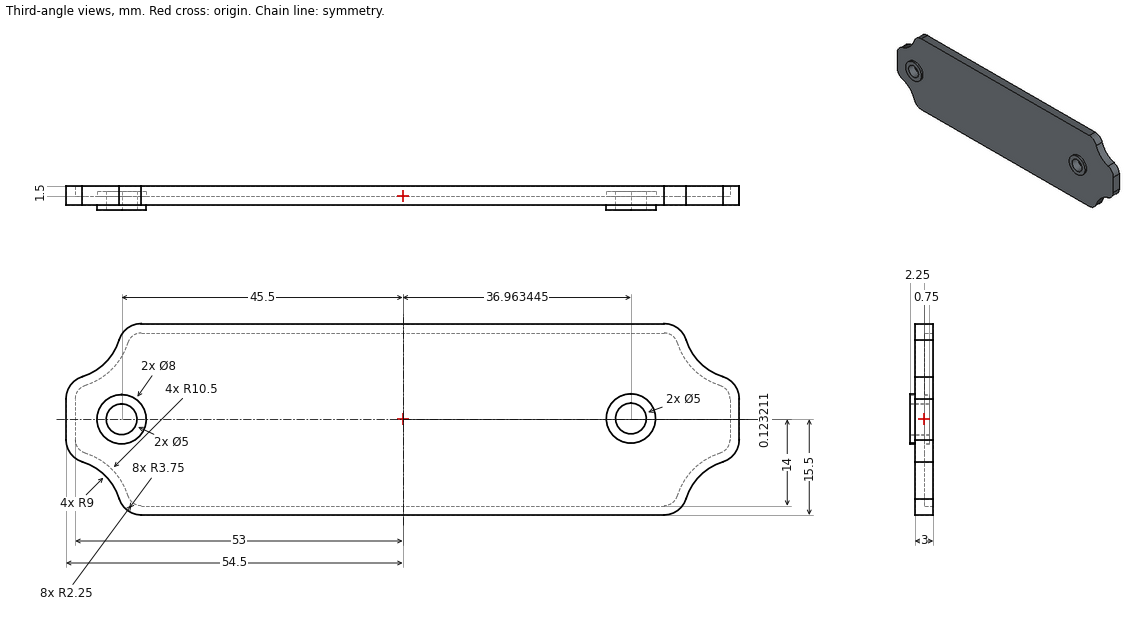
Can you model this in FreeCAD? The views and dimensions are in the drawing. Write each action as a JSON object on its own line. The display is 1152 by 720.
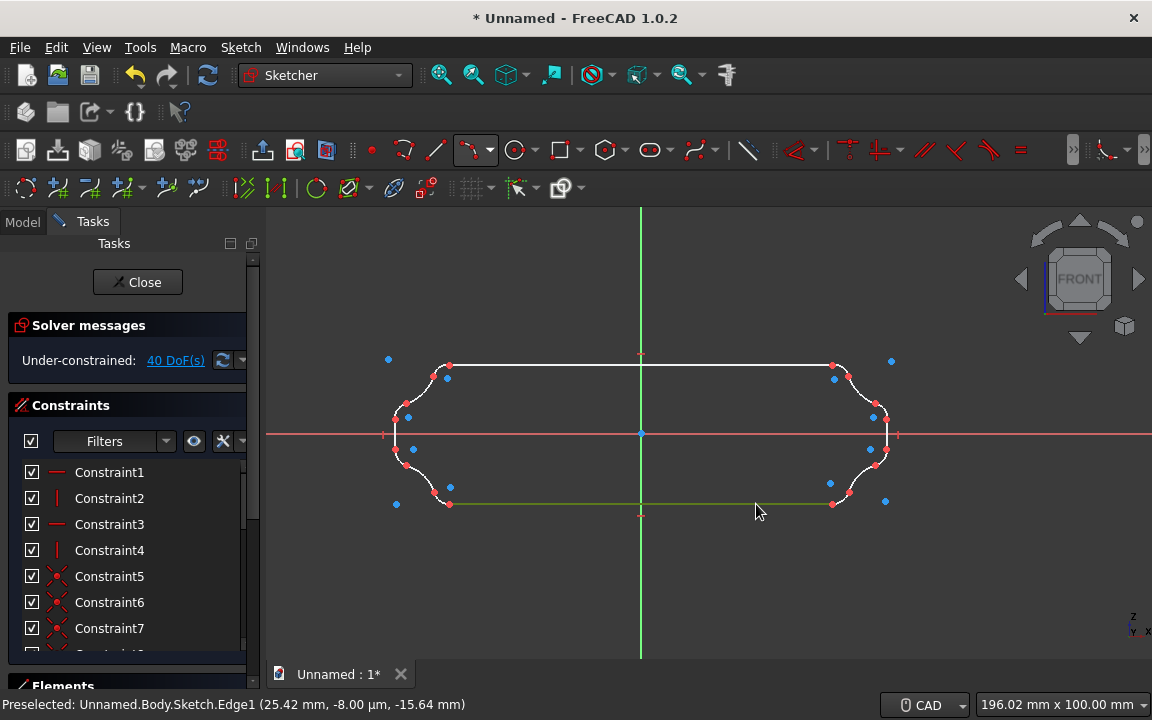
{"action": "scroll", "coordinate": [440, 501], "scroll_direction": "up", "scroll_amount": 2}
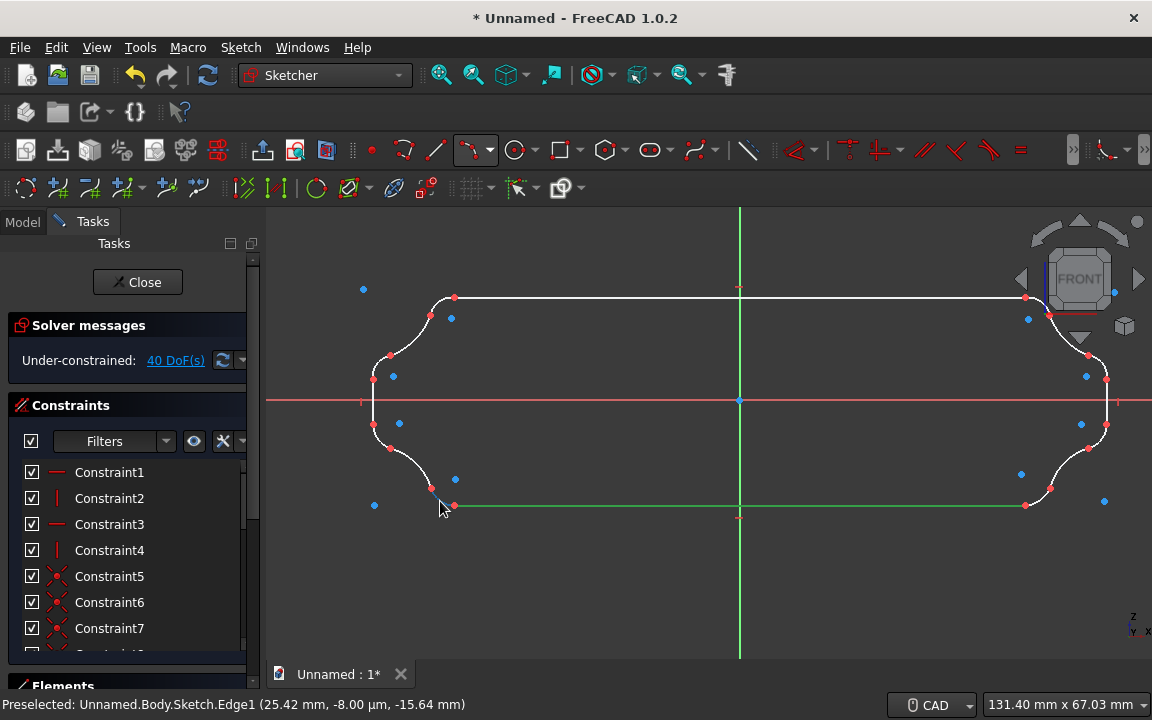
{"action": "left_click", "coordinate": [440, 501]}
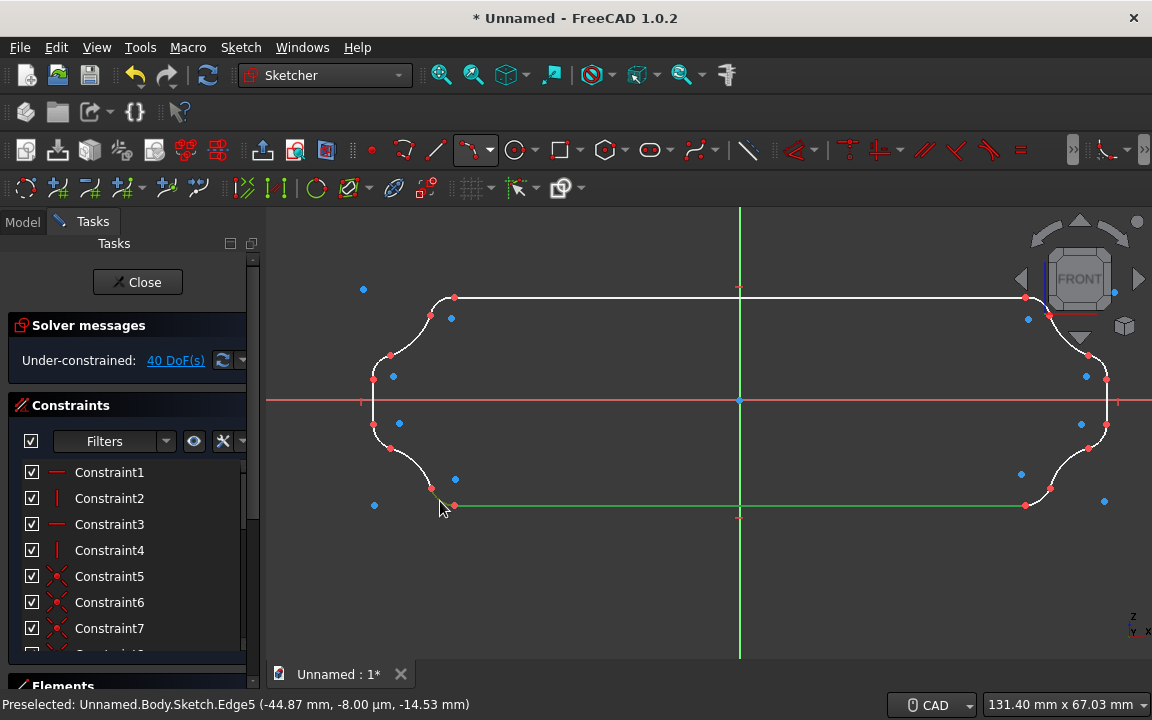
{"action": "left_click", "coordinate": [990, 150]}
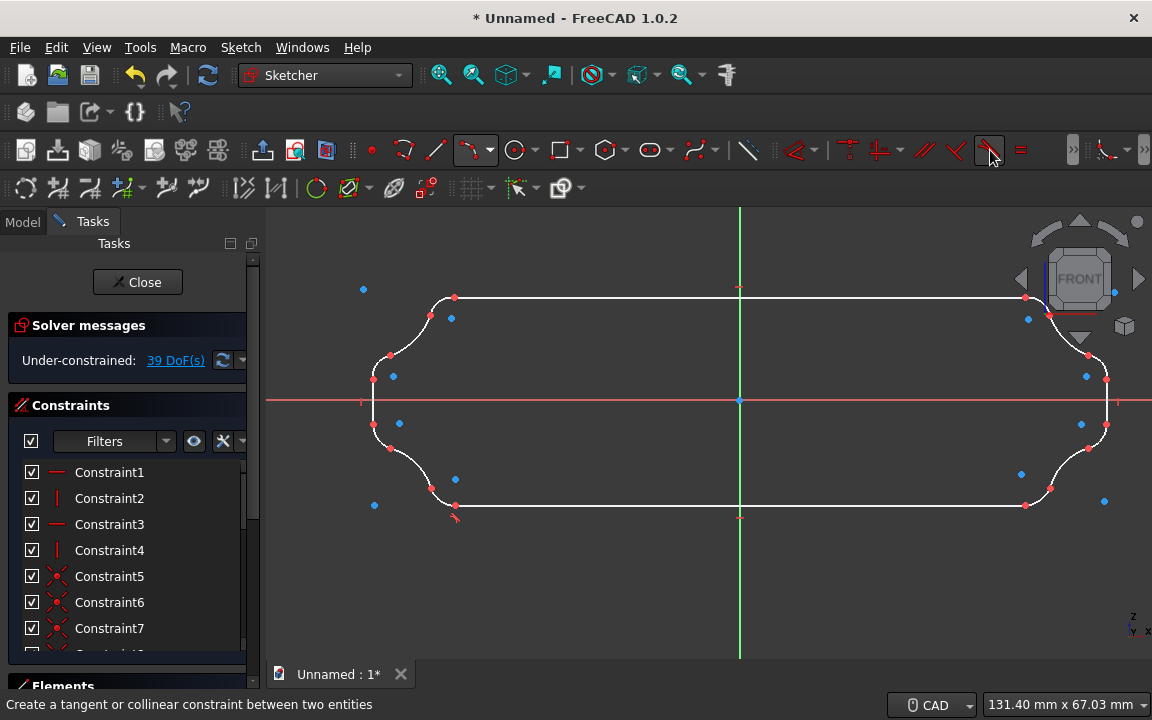
{"action": "left_click", "coordinate": [854, 506]}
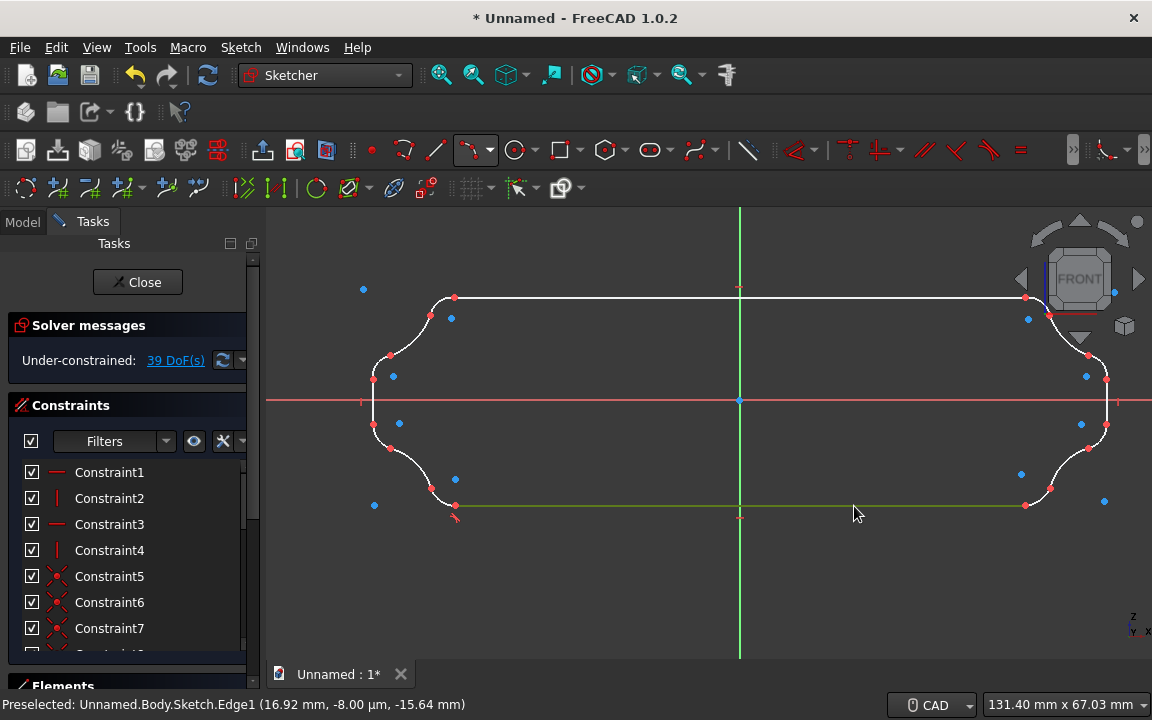
{"action": "scroll", "coordinate": [438, 499], "scroll_direction": "down", "scroll_amount": 2}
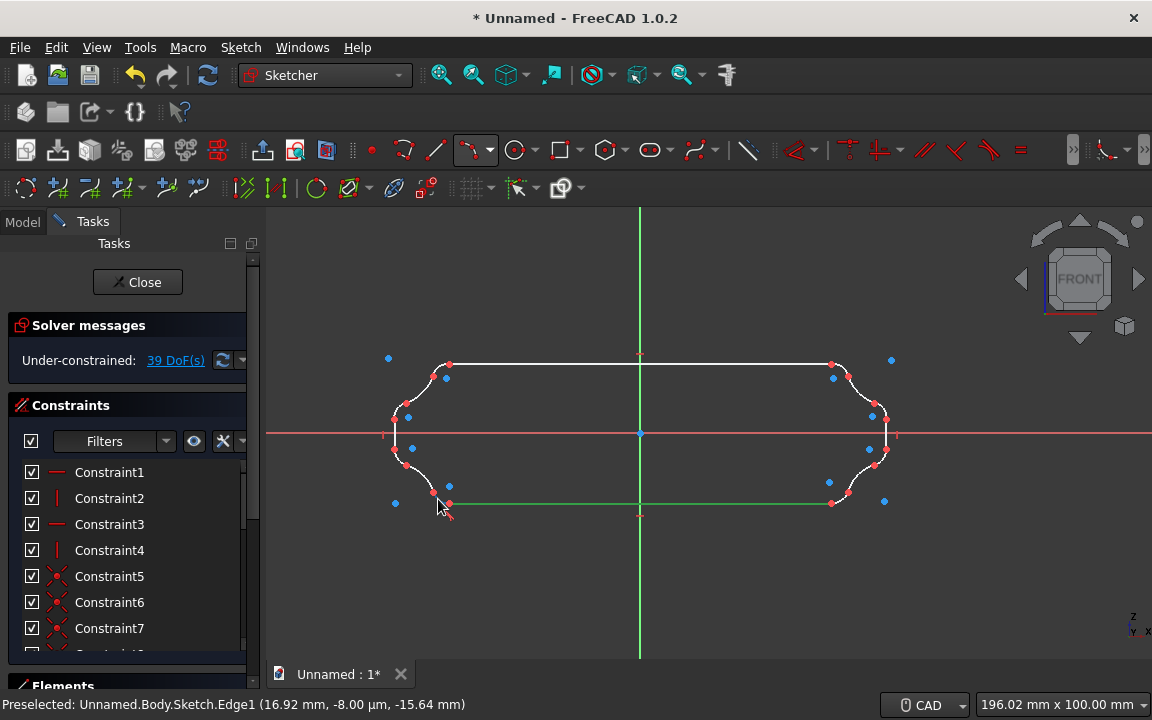
{"action": "scroll", "coordinate": [838, 502], "scroll_direction": "up", "scroll_amount": 4}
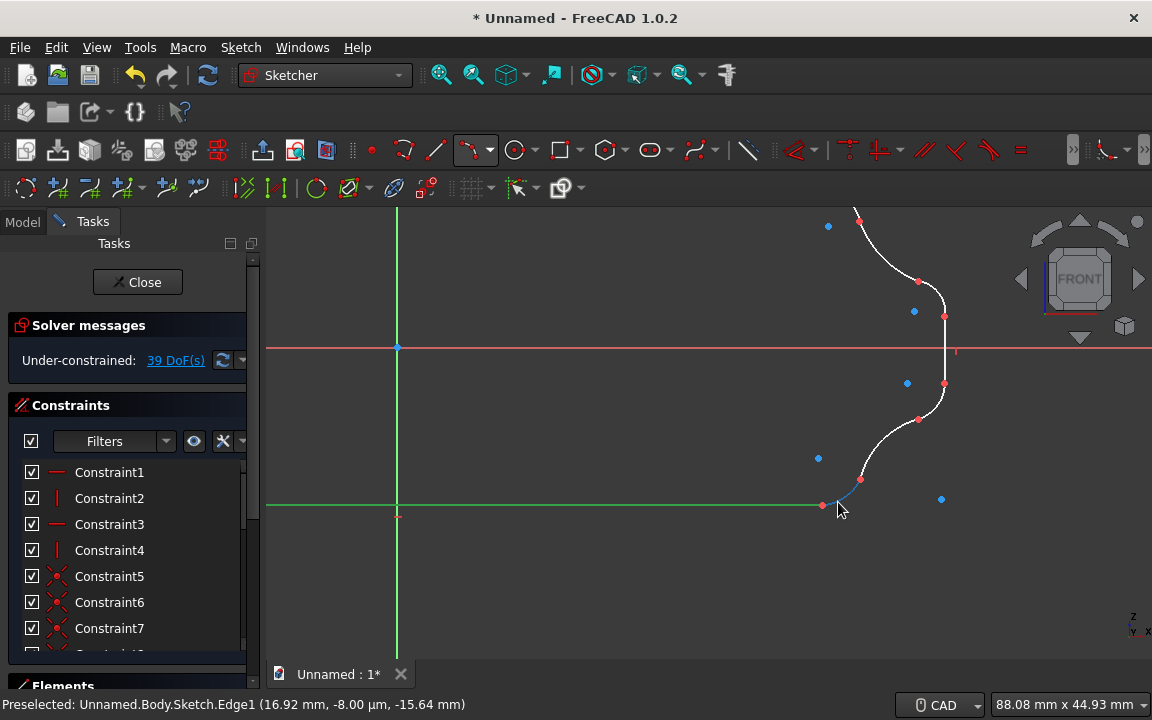
{"action": "left_click", "coordinate": [837, 502]}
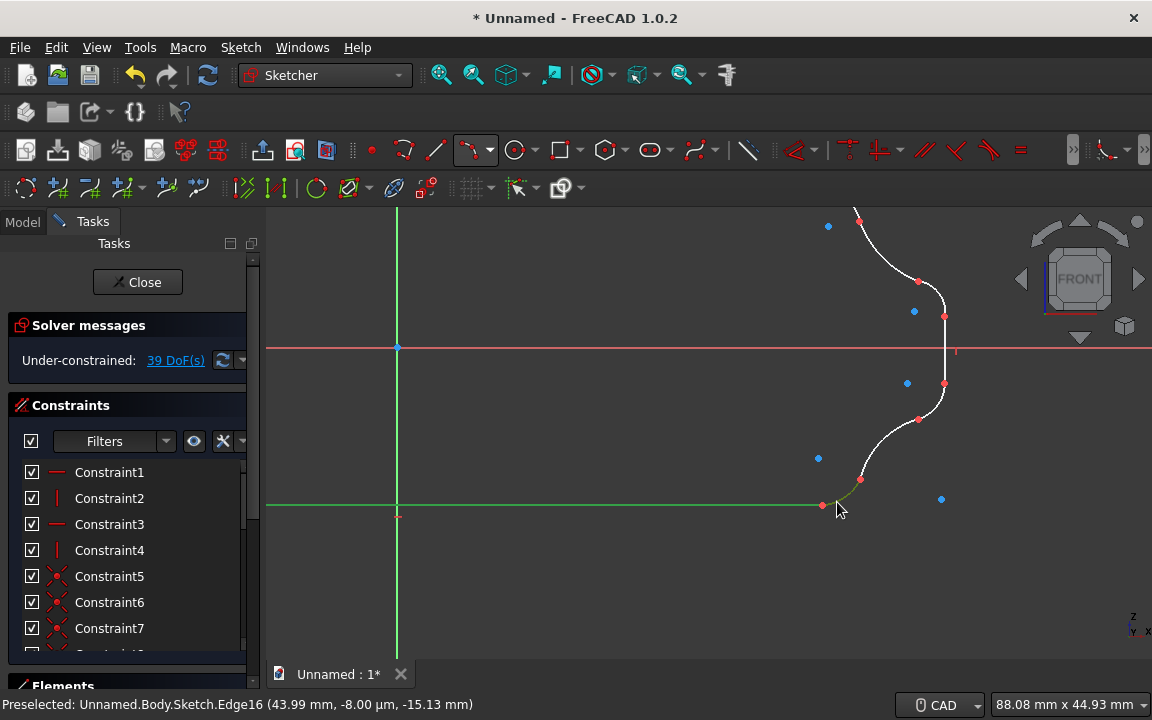
{"action": "left_click", "coordinate": [990, 150]}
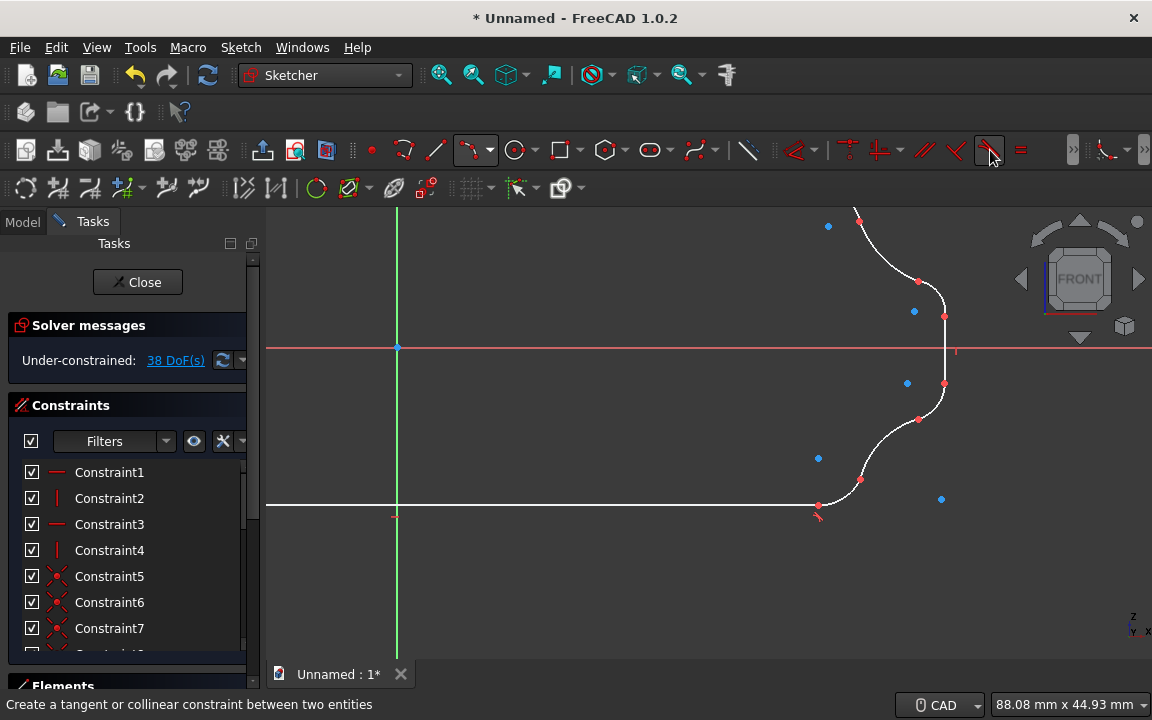
{"action": "scroll", "coordinate": [839, 502], "scroll_direction": "down", "scroll_amount": 4}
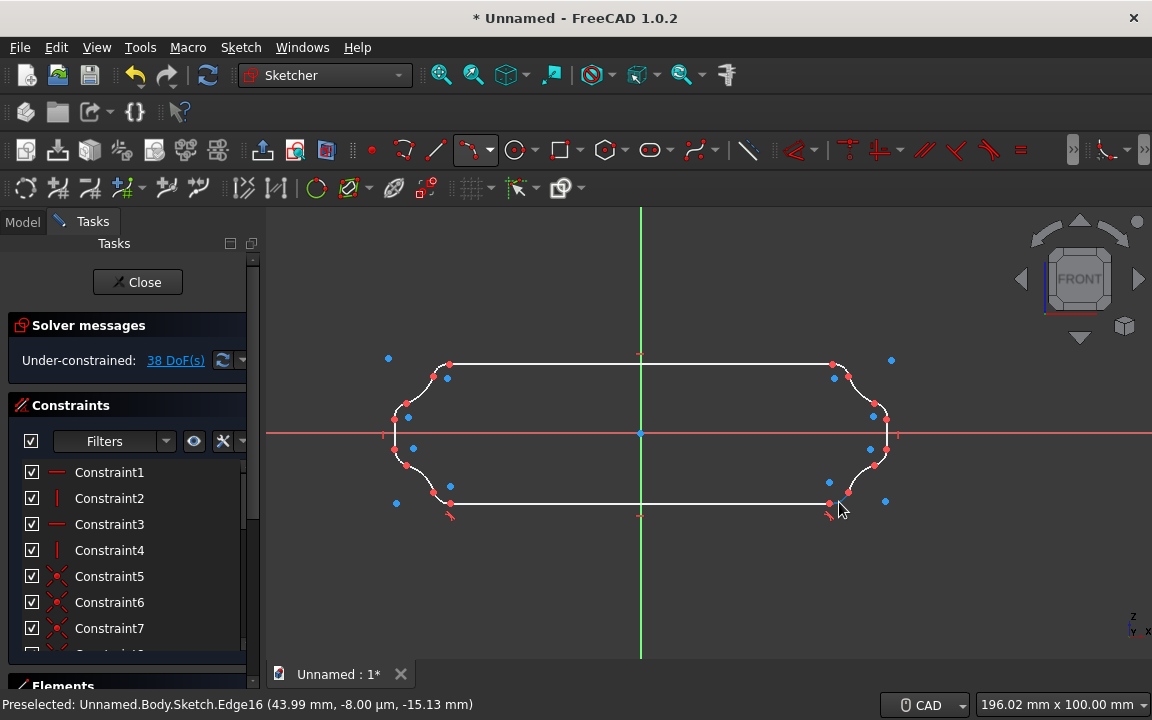
{"action": "scroll", "coordinate": [395, 440], "scroll_direction": "up", "scroll_amount": 4}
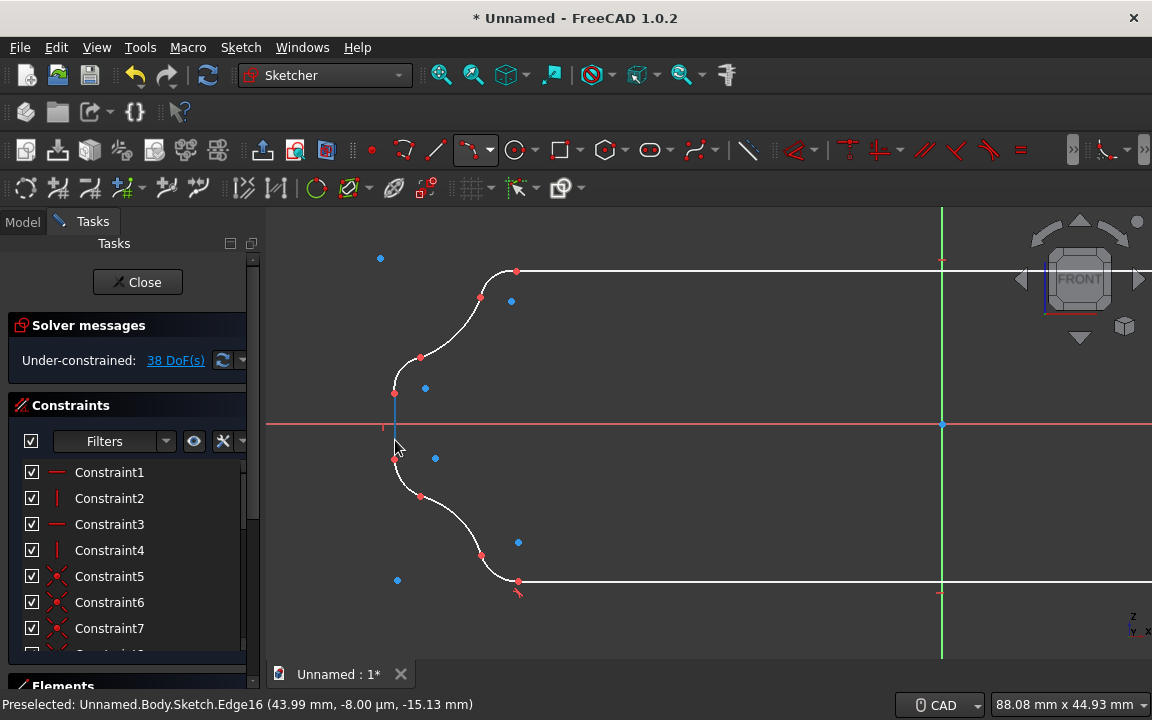
{"action": "left_click", "coordinate": [395, 440]}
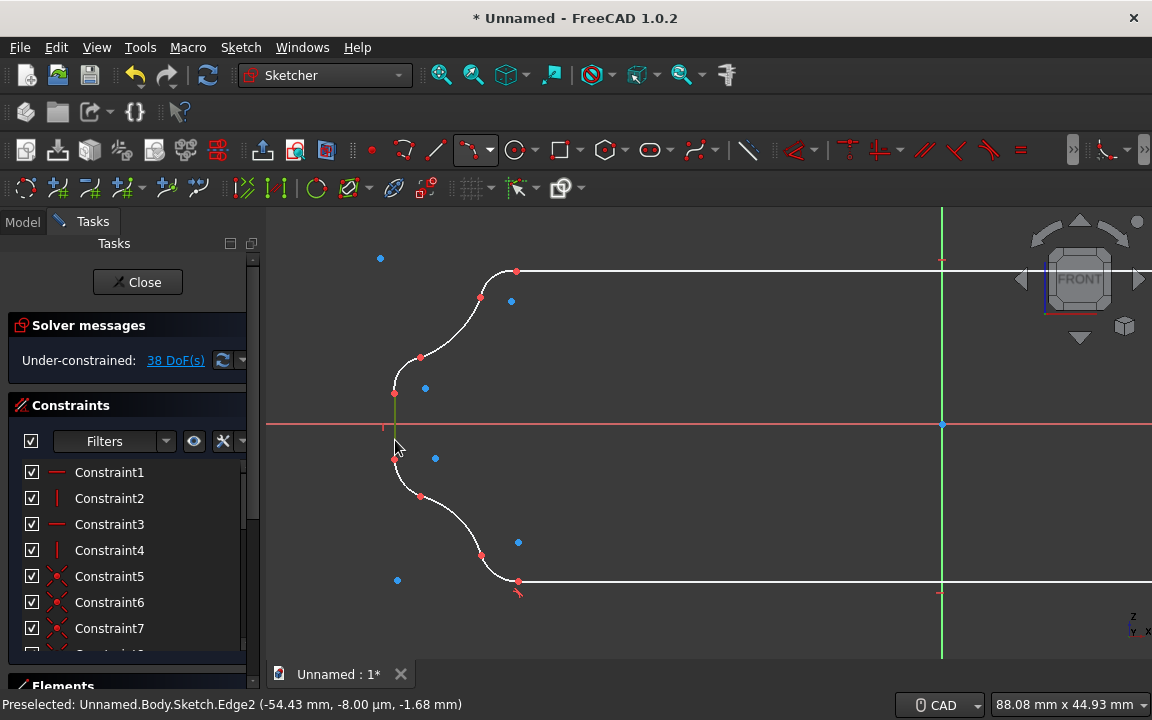
{"action": "left_click", "coordinate": [398, 473]}